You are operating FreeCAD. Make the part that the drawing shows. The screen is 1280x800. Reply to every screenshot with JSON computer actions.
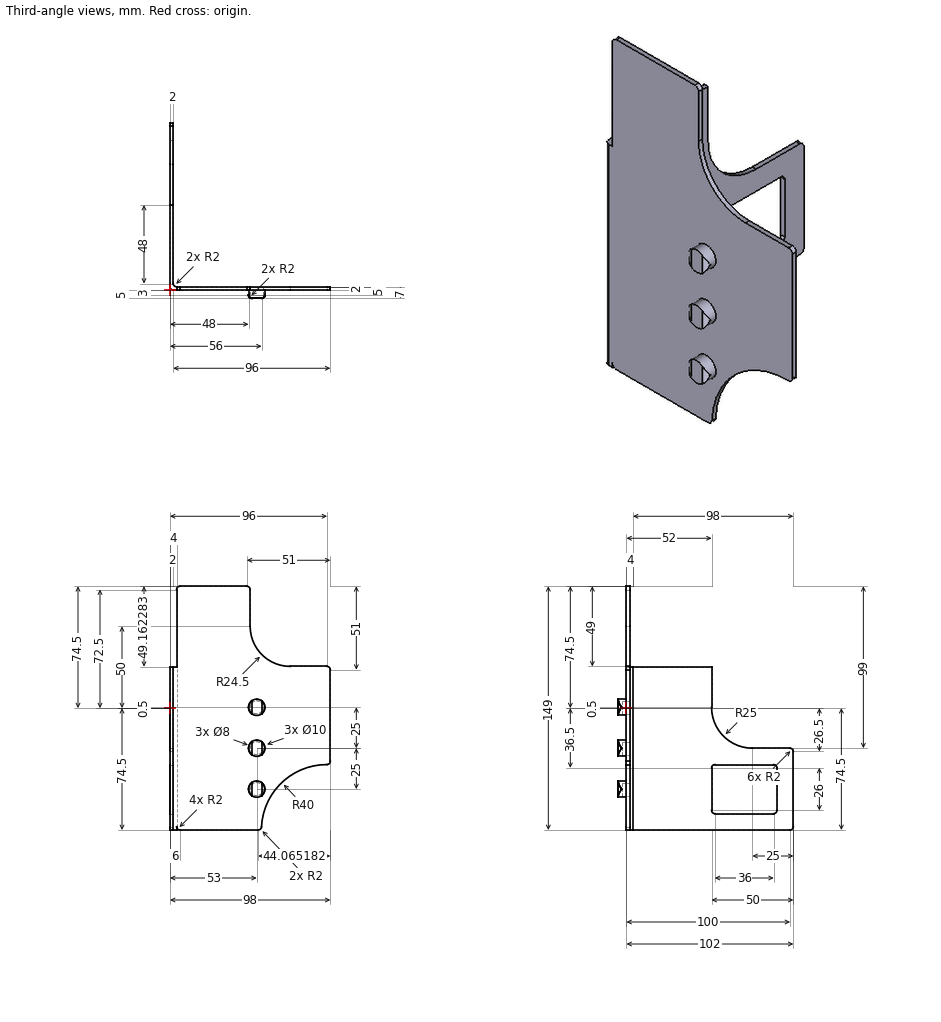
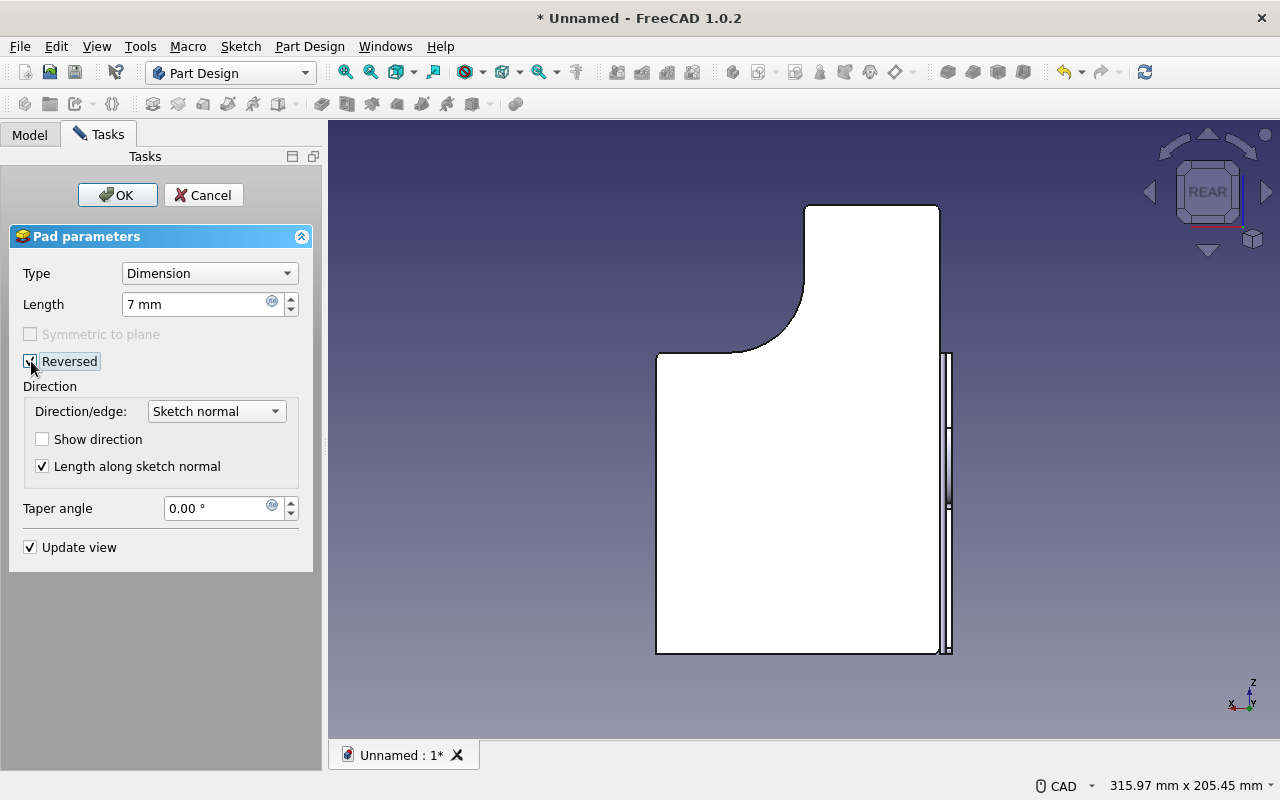
{"action": "left_click", "coordinate": [118, 195]}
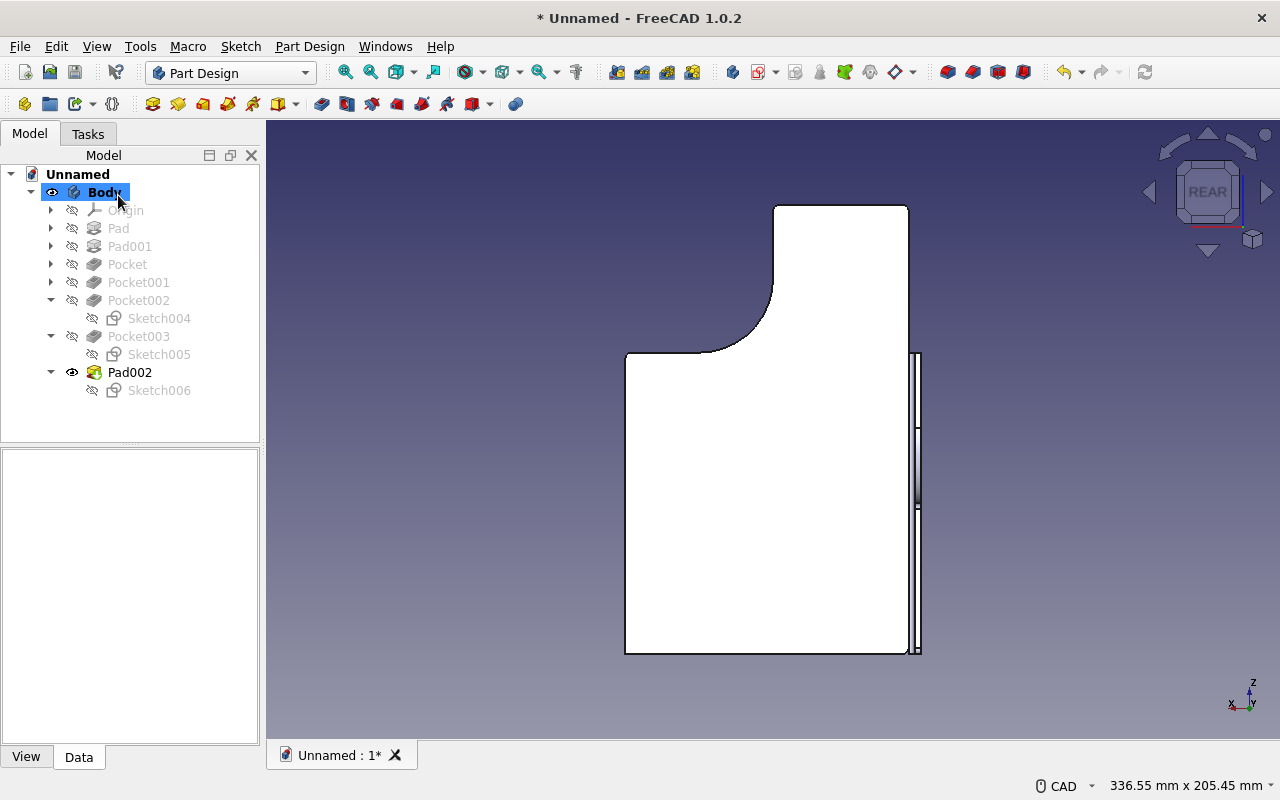
{"action": "left_click", "coordinate": [758, 72]}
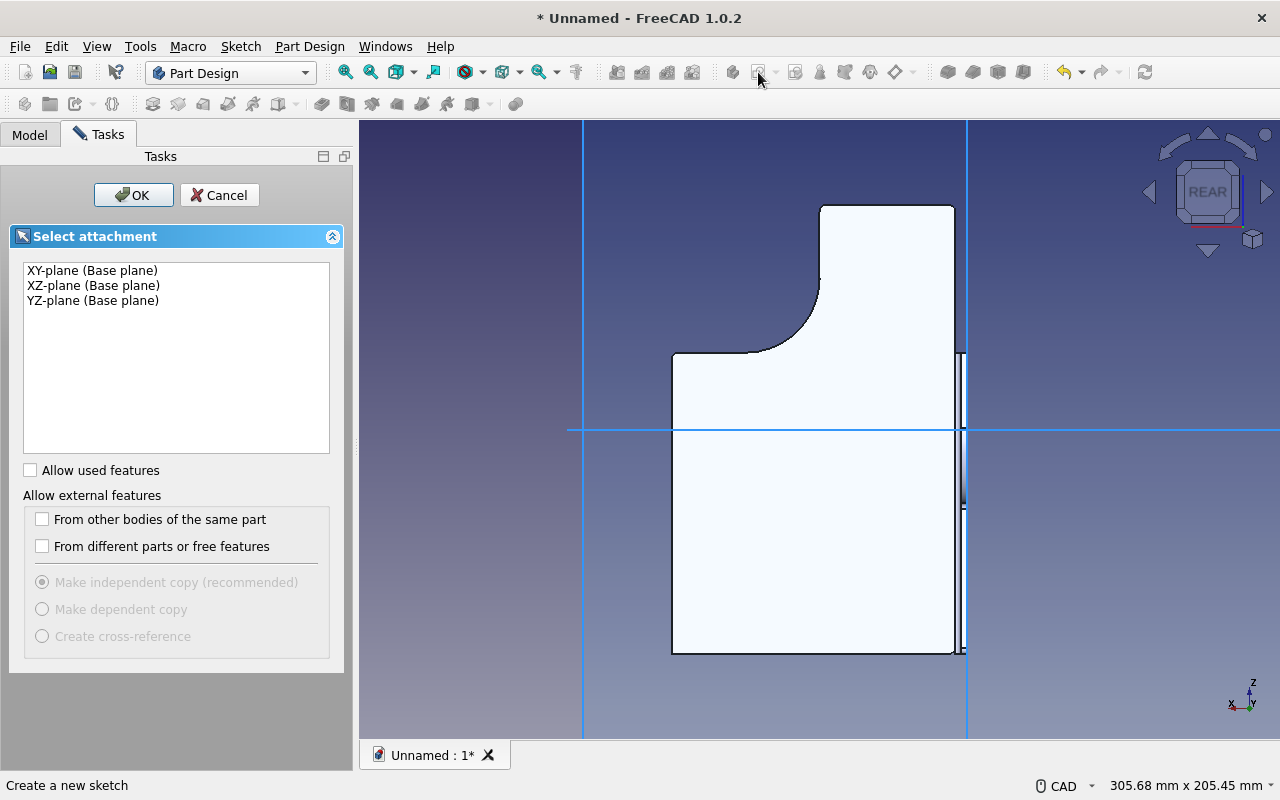
{"action": "left_click", "coordinate": [84, 270]}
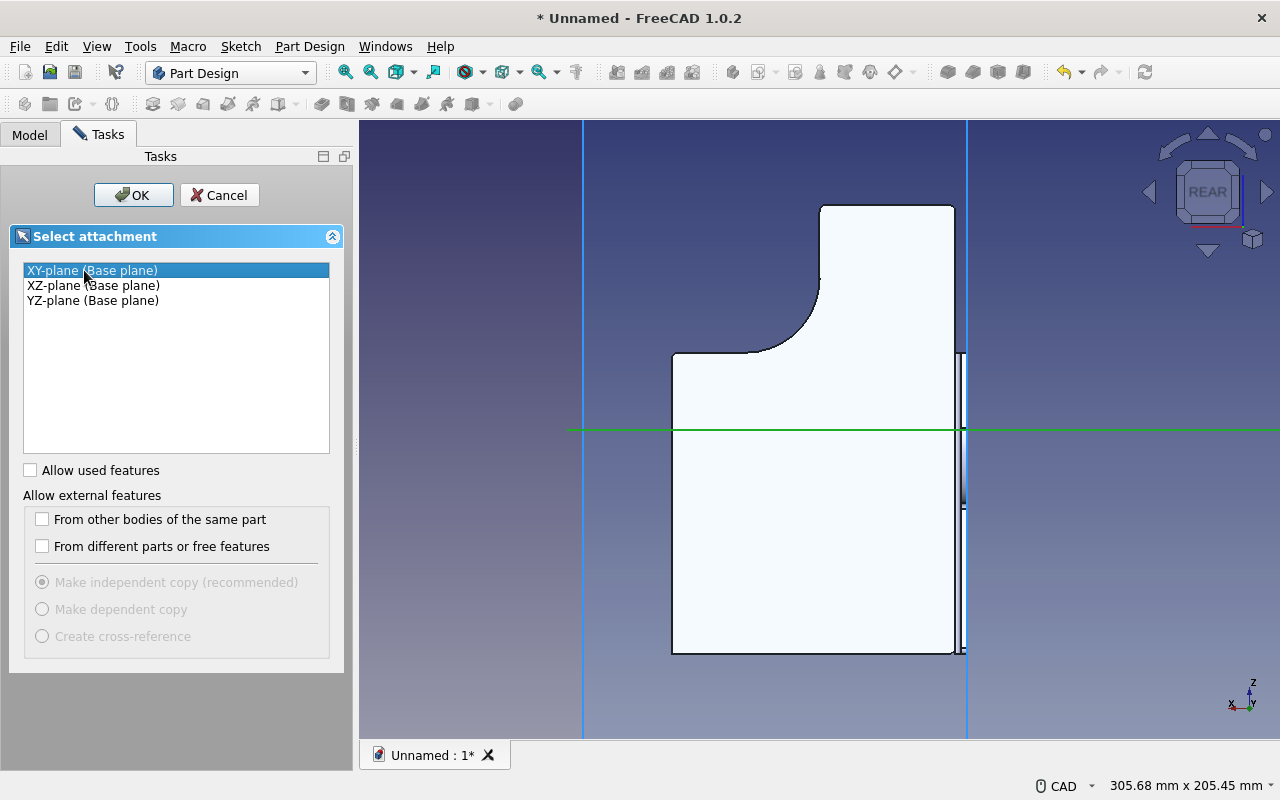
{"action": "left_click", "coordinate": [134, 195]}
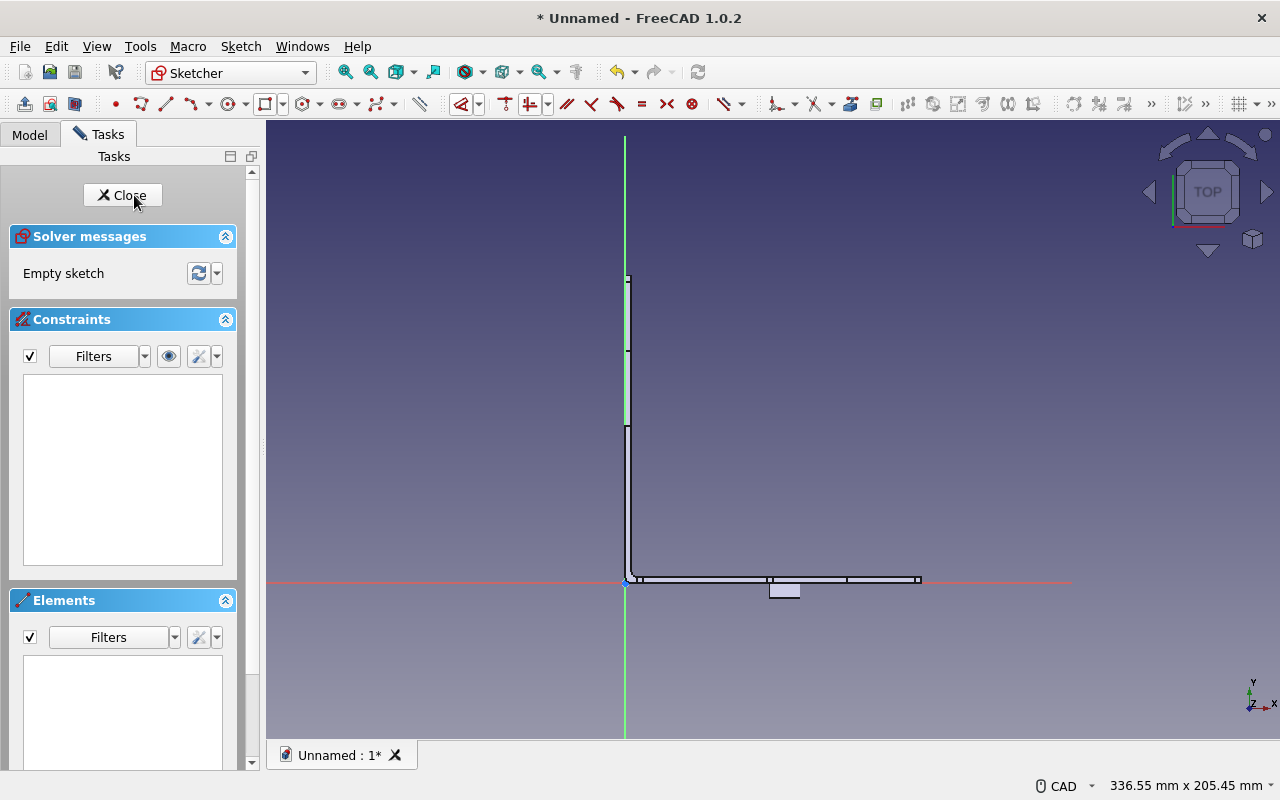
{"action": "key", "text": "q s"}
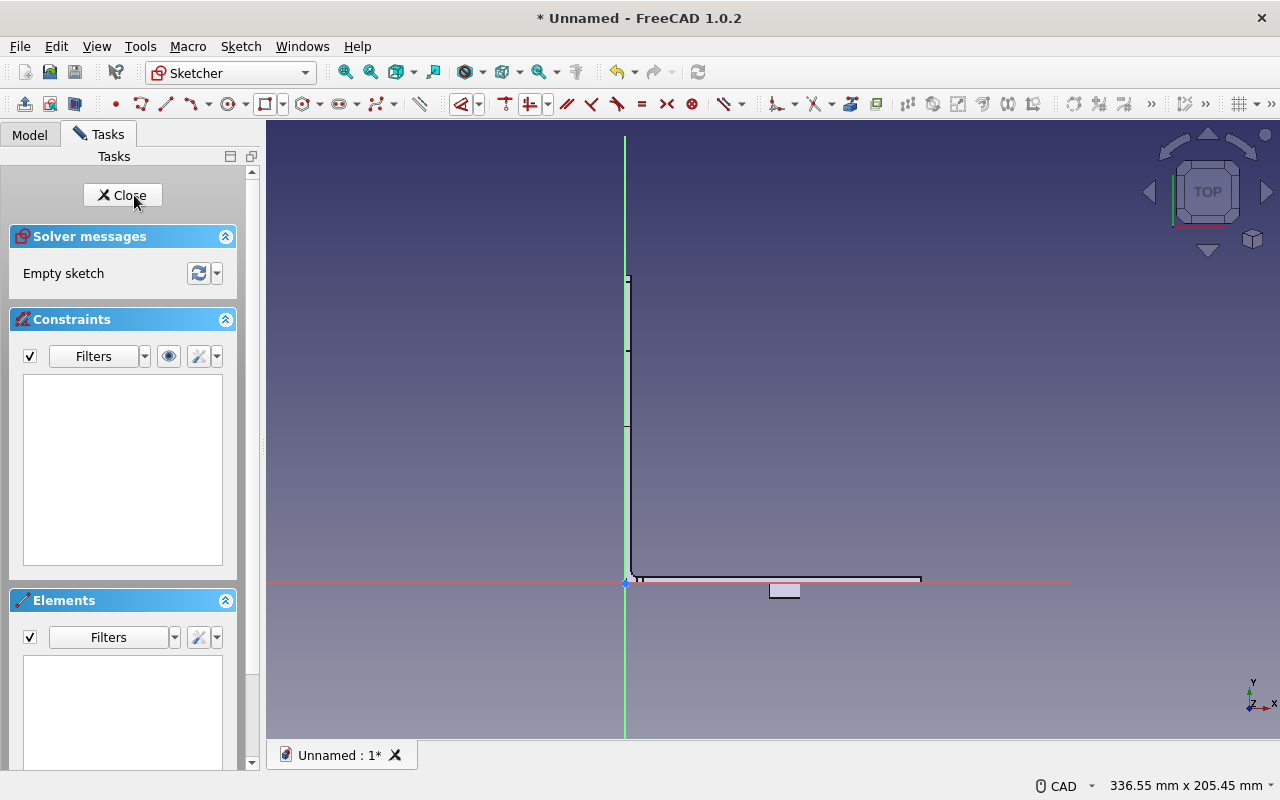
{"action": "scroll", "coordinate": [789, 604], "scroll_direction": "up", "scroll_amount": 15}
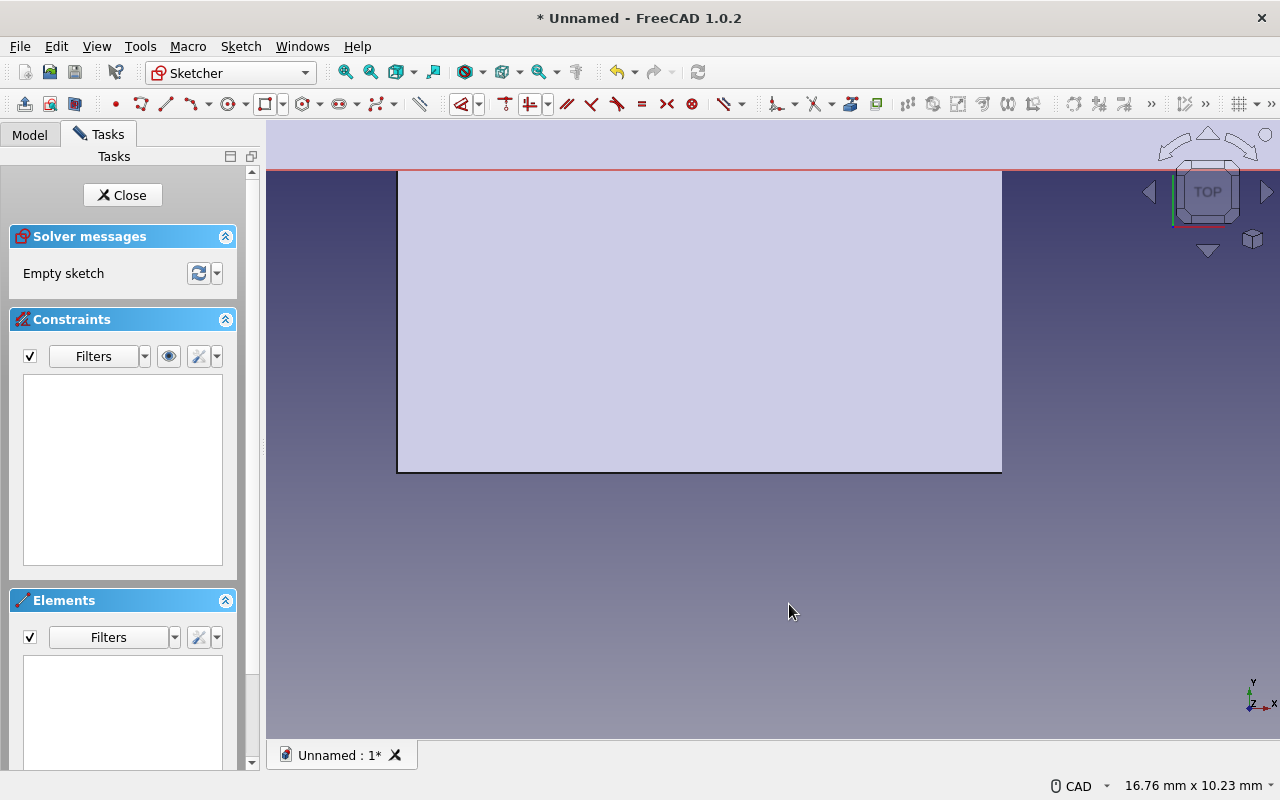
{"action": "left_click", "coordinate": [141, 104]}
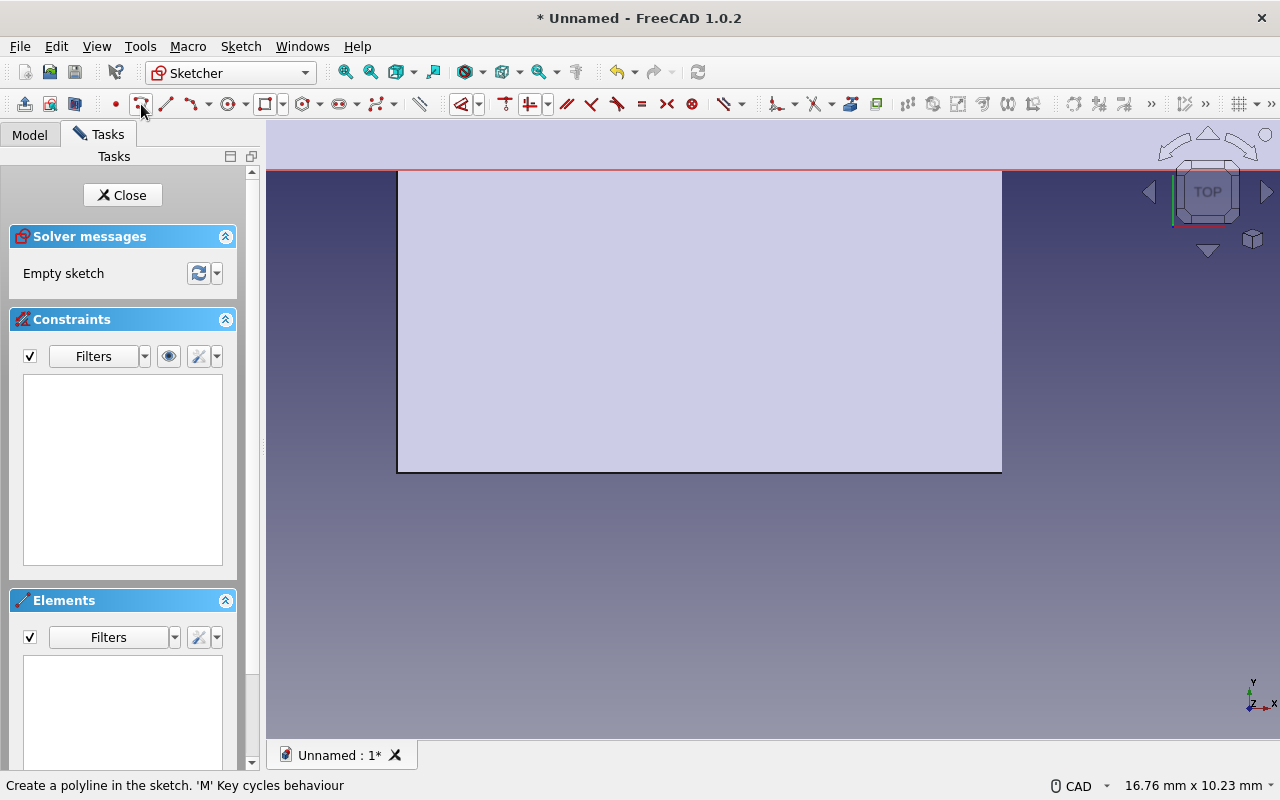
{"action": "left_click", "coordinate": [397, 352]}
{"action": "left_click", "coordinate": [397, 473]}
{"action": "left_click", "coordinate": [518, 473]}
{"action": "right_click", "coordinate": [518, 473]}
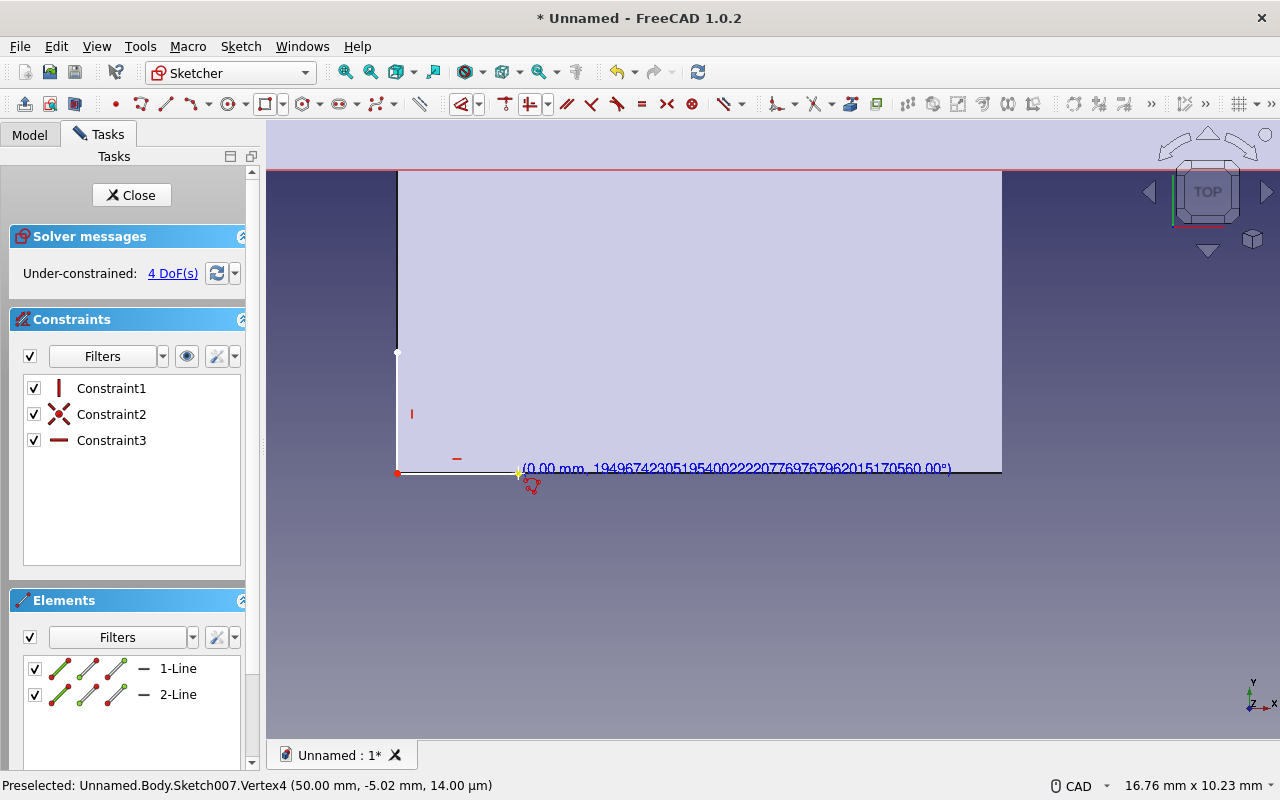
{"action": "key", "text": "g 3 a"}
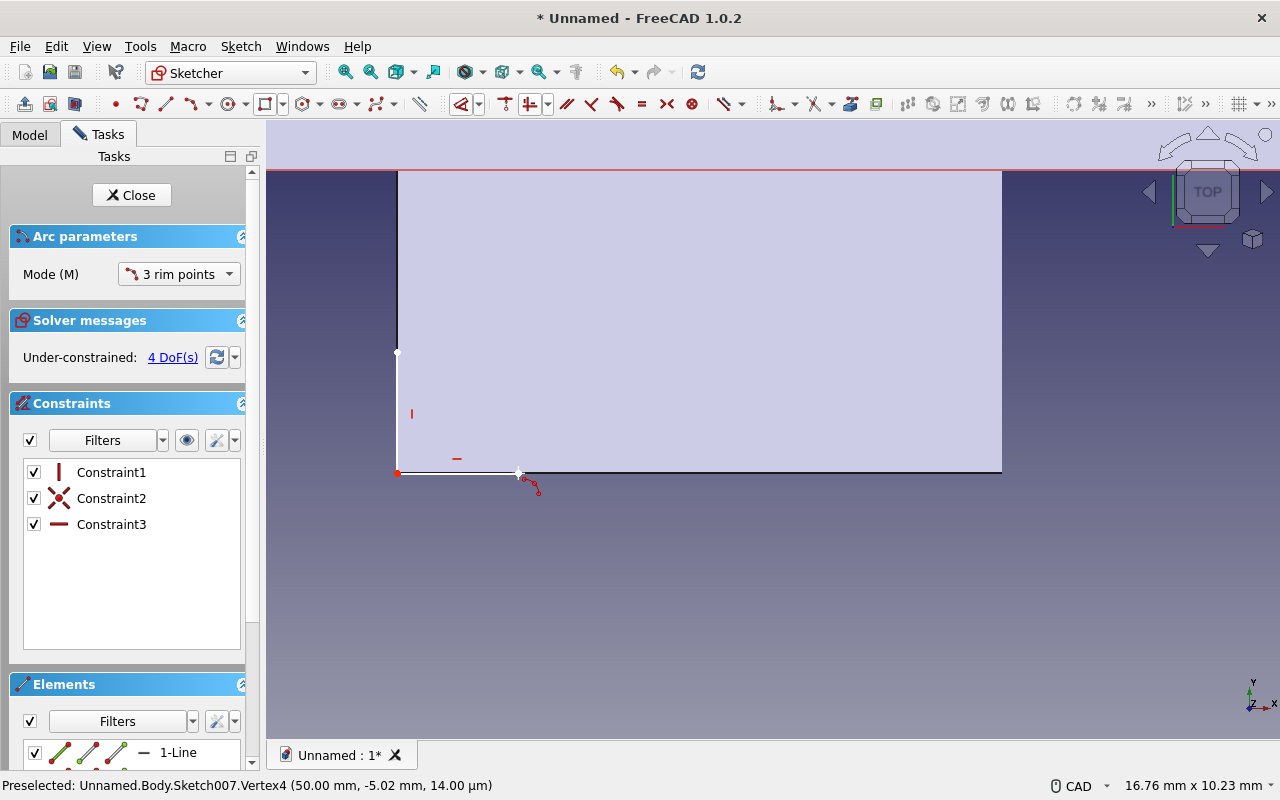
{"action": "left_click", "coordinate": [518, 474]}
{"action": "left_click", "coordinate": [397, 353]}
{"action": "left_click", "coordinate": [433, 438]}